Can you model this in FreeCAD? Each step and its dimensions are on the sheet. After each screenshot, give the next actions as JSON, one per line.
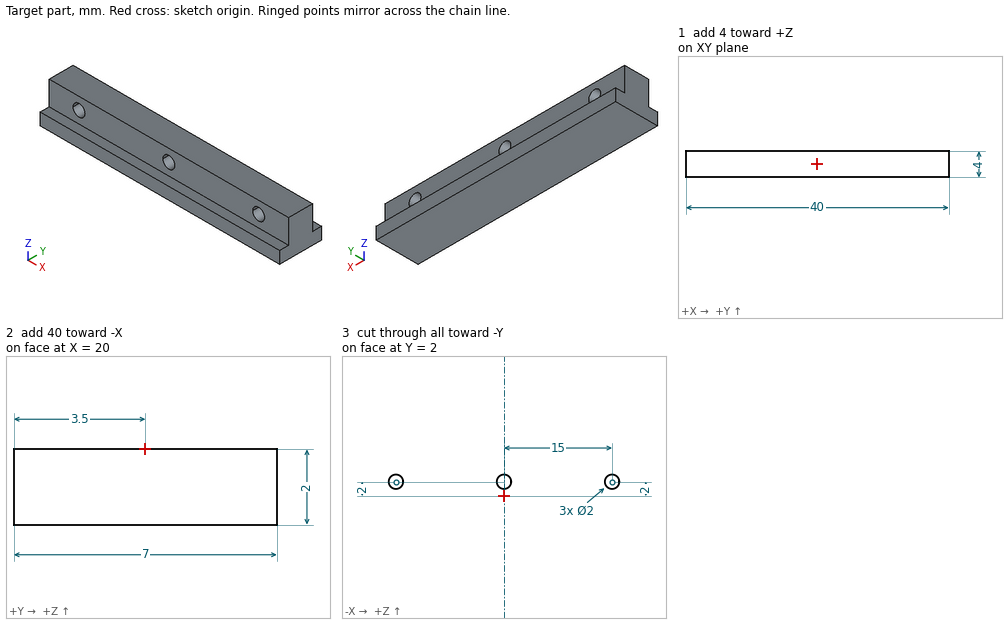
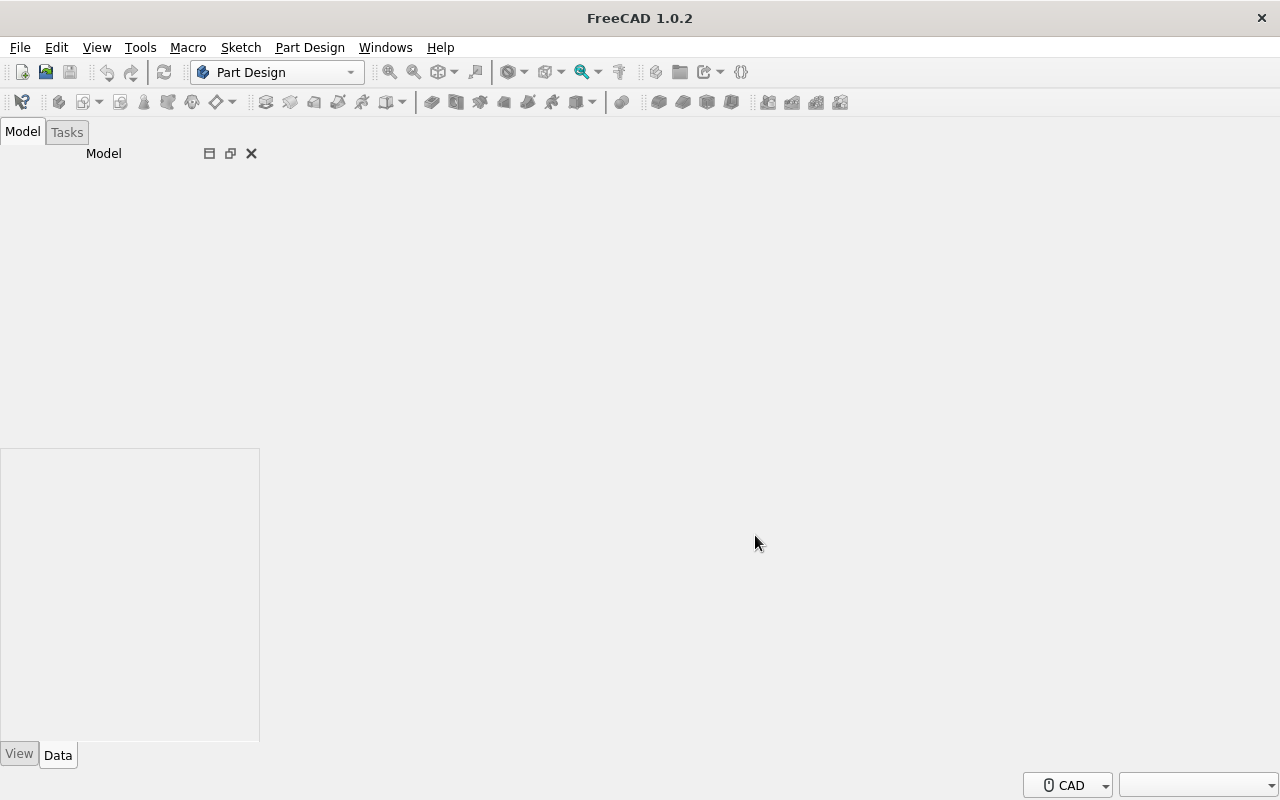
{"action": "key", "text": "ctrl+n"}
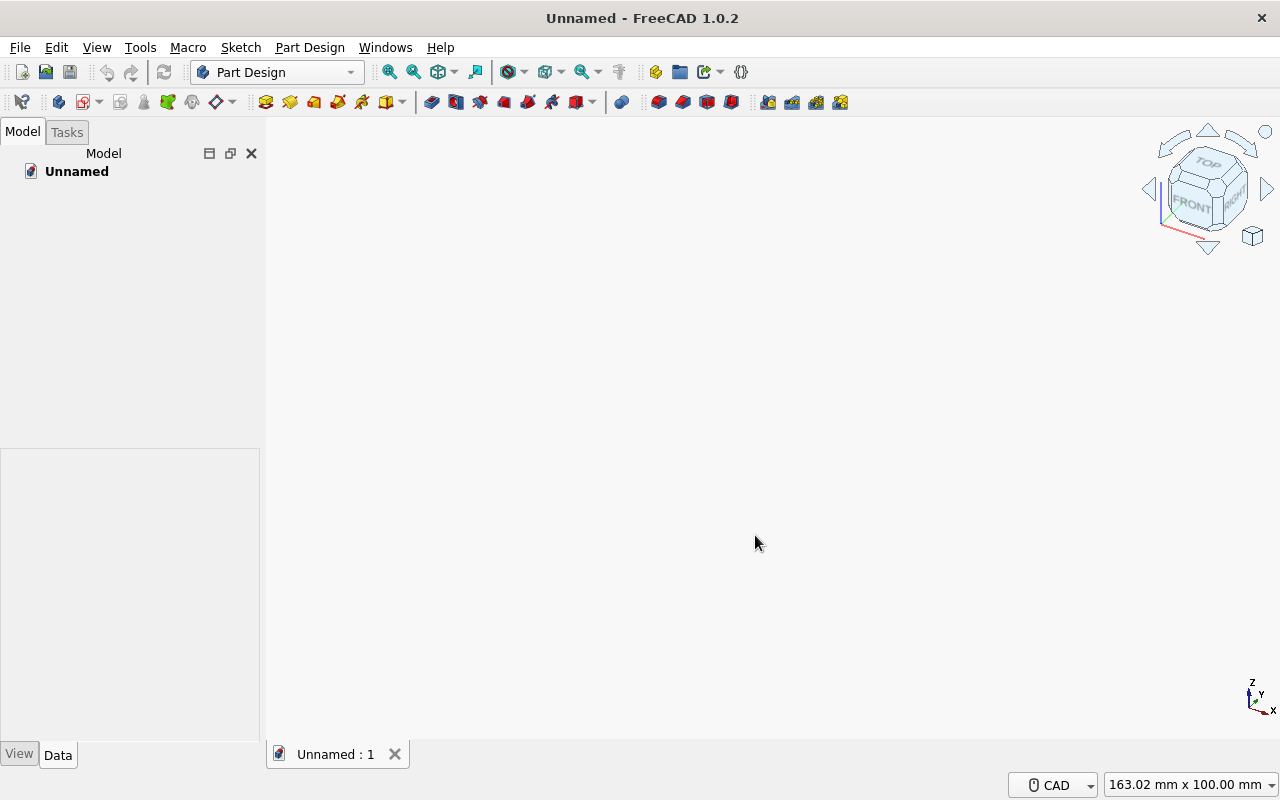
{"action": "left_click", "coordinate": [84, 102]}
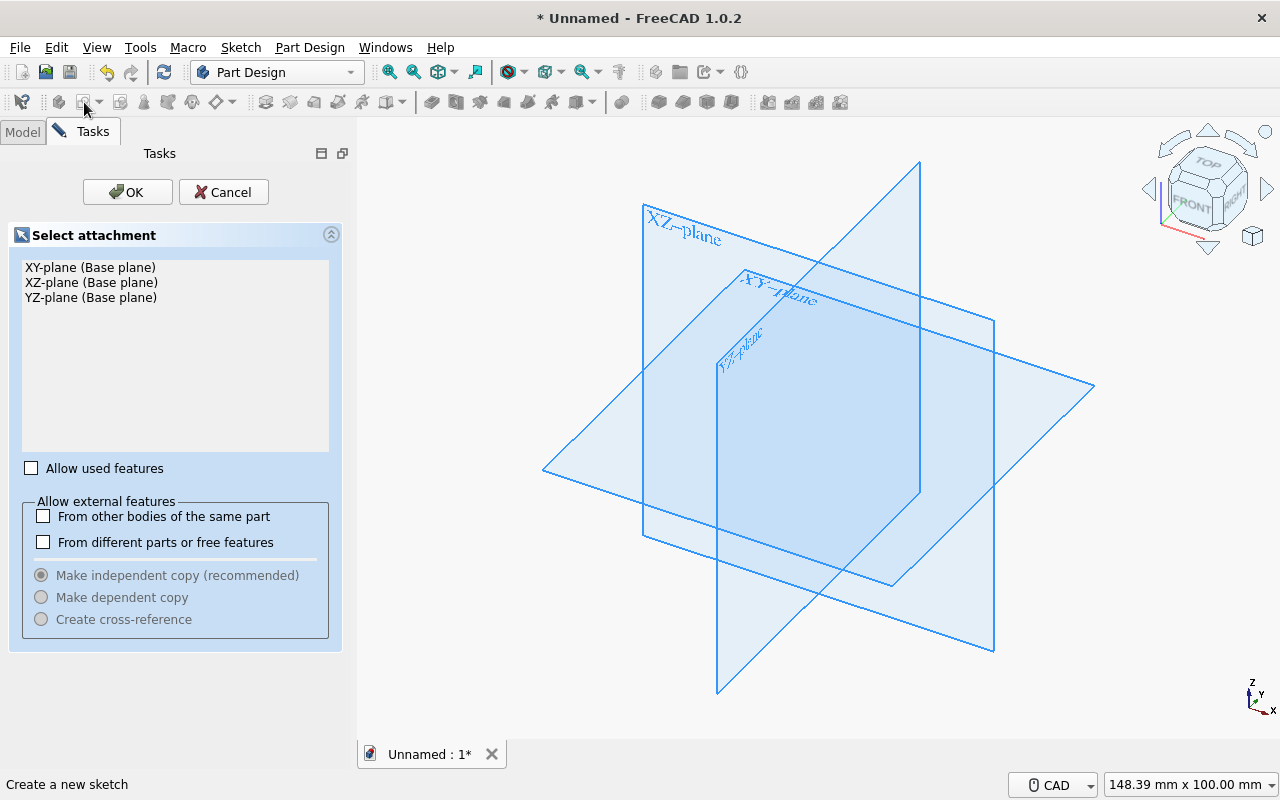
{"action": "left_click", "coordinate": [82, 268]}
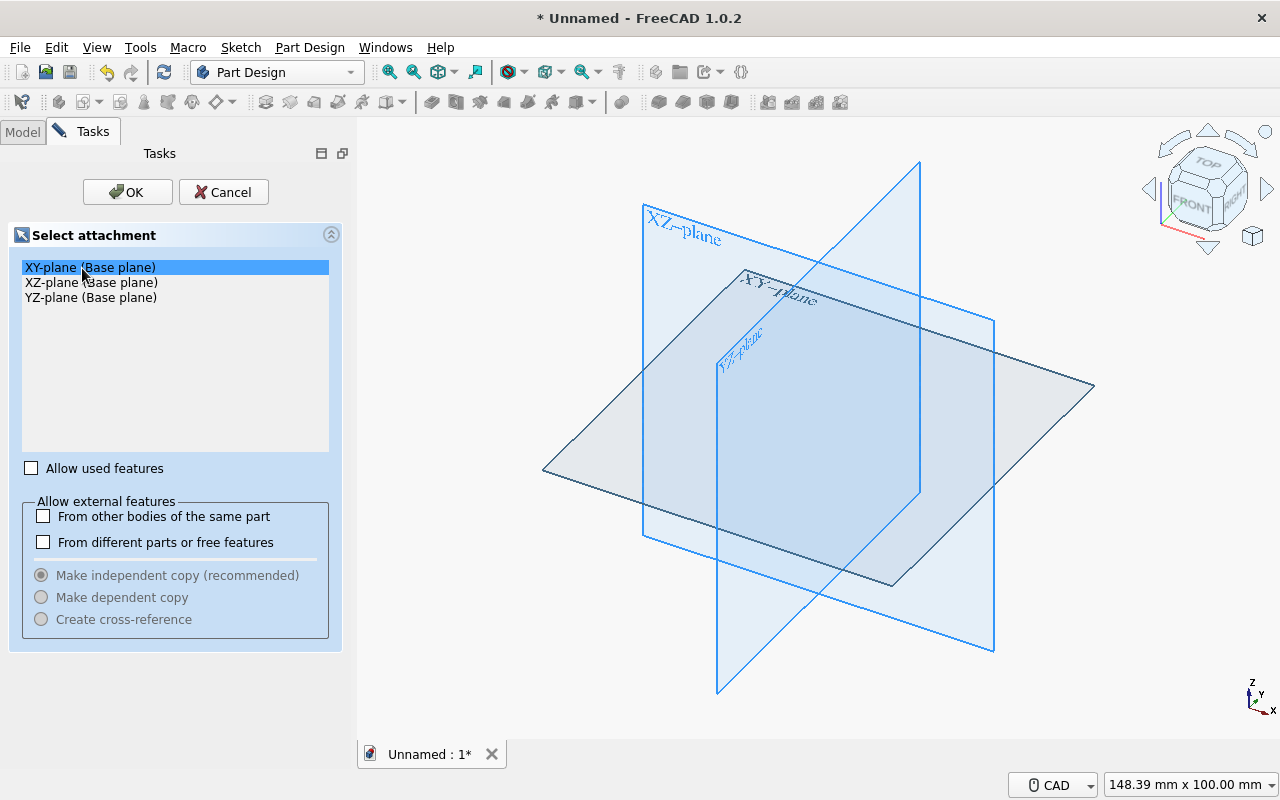
{"action": "left_click", "coordinate": [128, 192]}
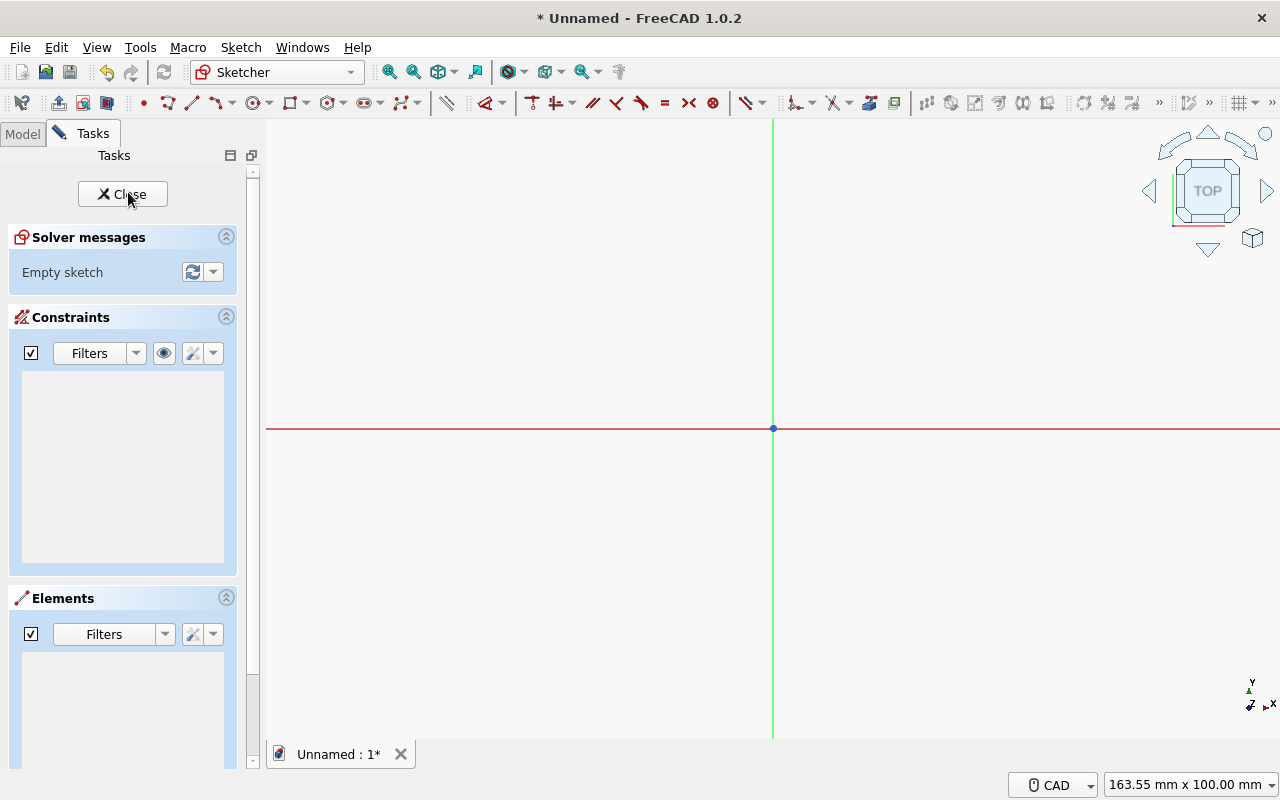
{"action": "scroll", "coordinate": [829, 429], "scroll_direction": "up", "scroll_amount": 4}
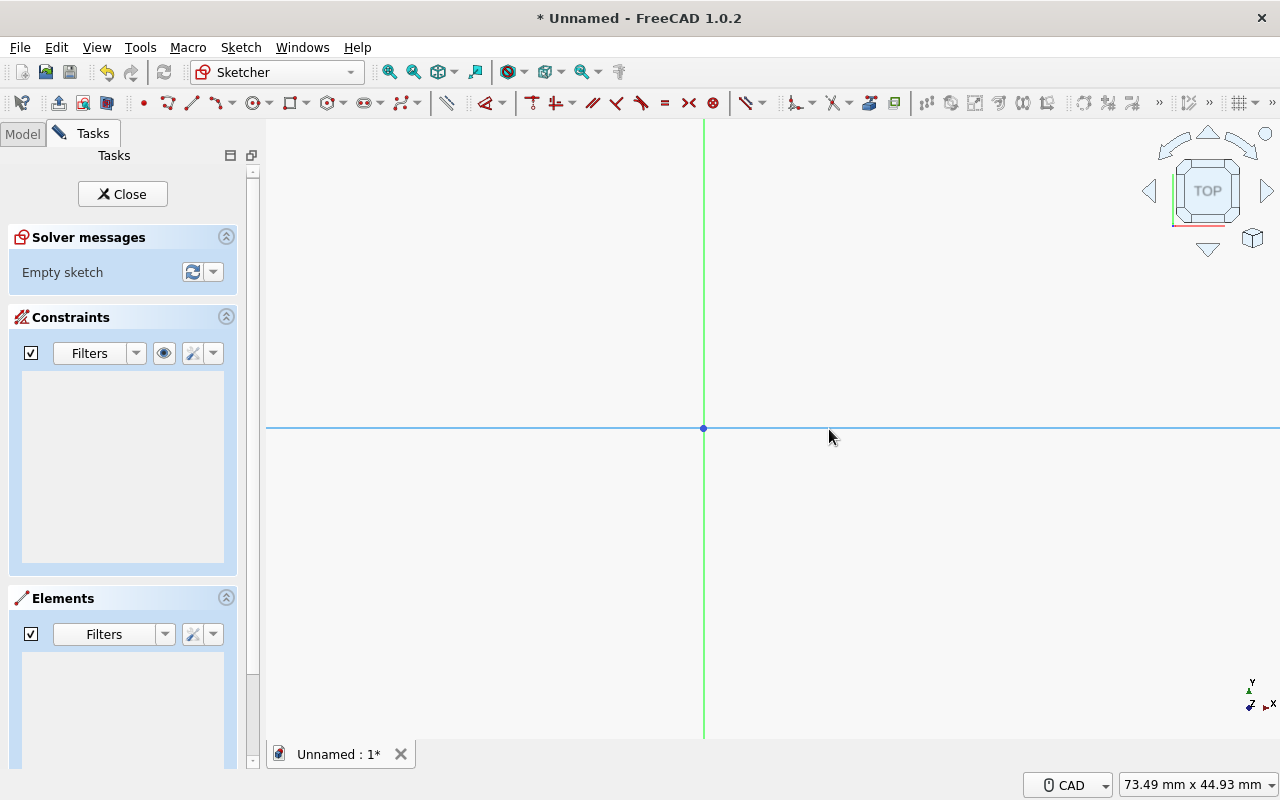
{"action": "left_click", "coordinate": [308, 104]}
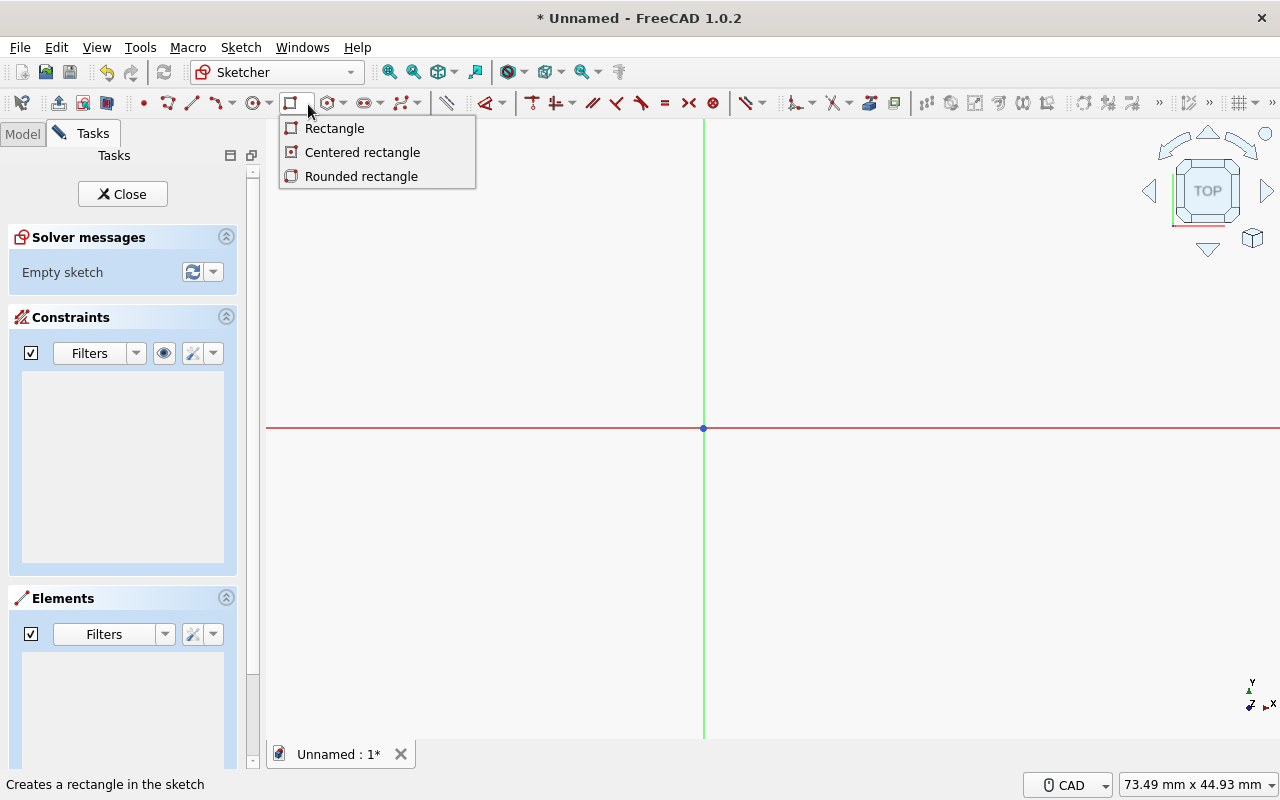
{"action": "left_click", "coordinate": [378, 152]}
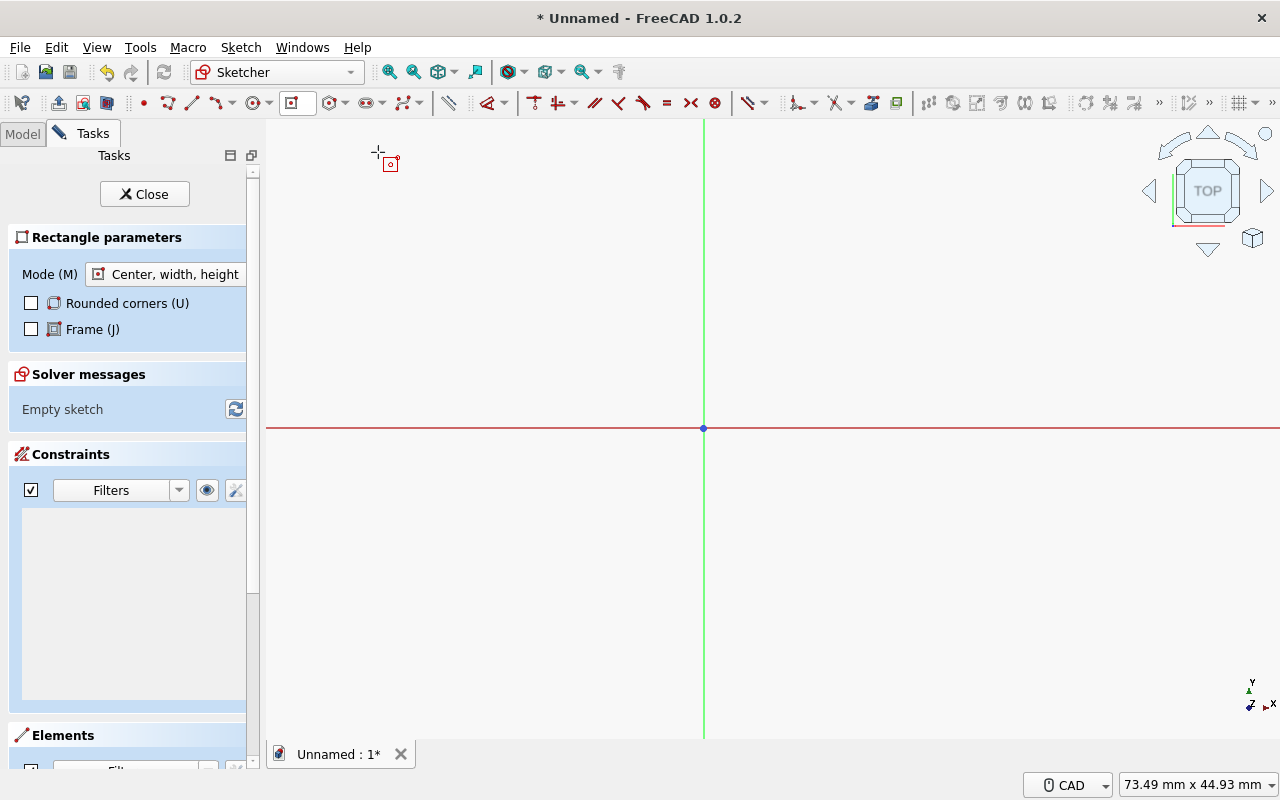
{"action": "left_click", "coordinate": [704, 428]}
{"action": "mouse_move", "coordinate": [980, 401]}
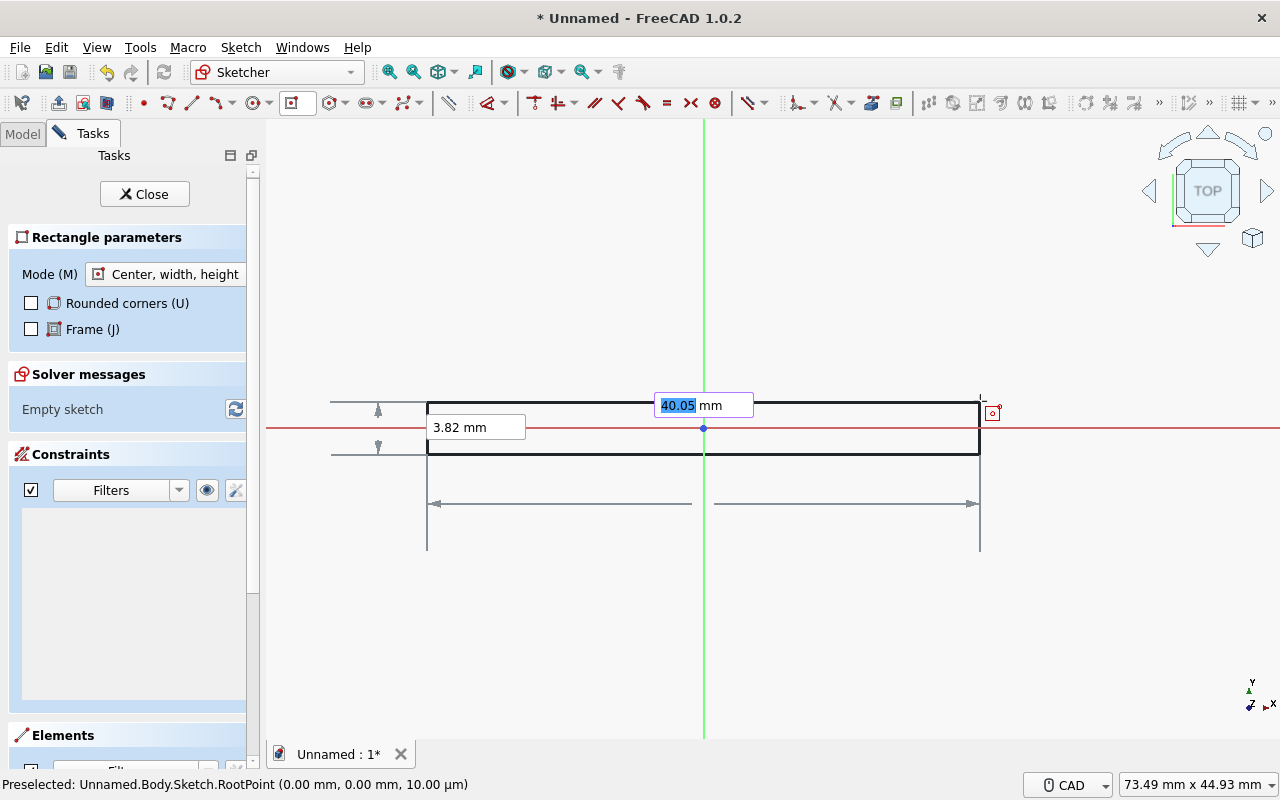
{"action": "type", "text": "40"}
{"action": "key", "text": "Tab"}
{"action": "type", "text": "4"}
{"action": "key", "text": "Return"}
{"action": "key", "text": "Escape"}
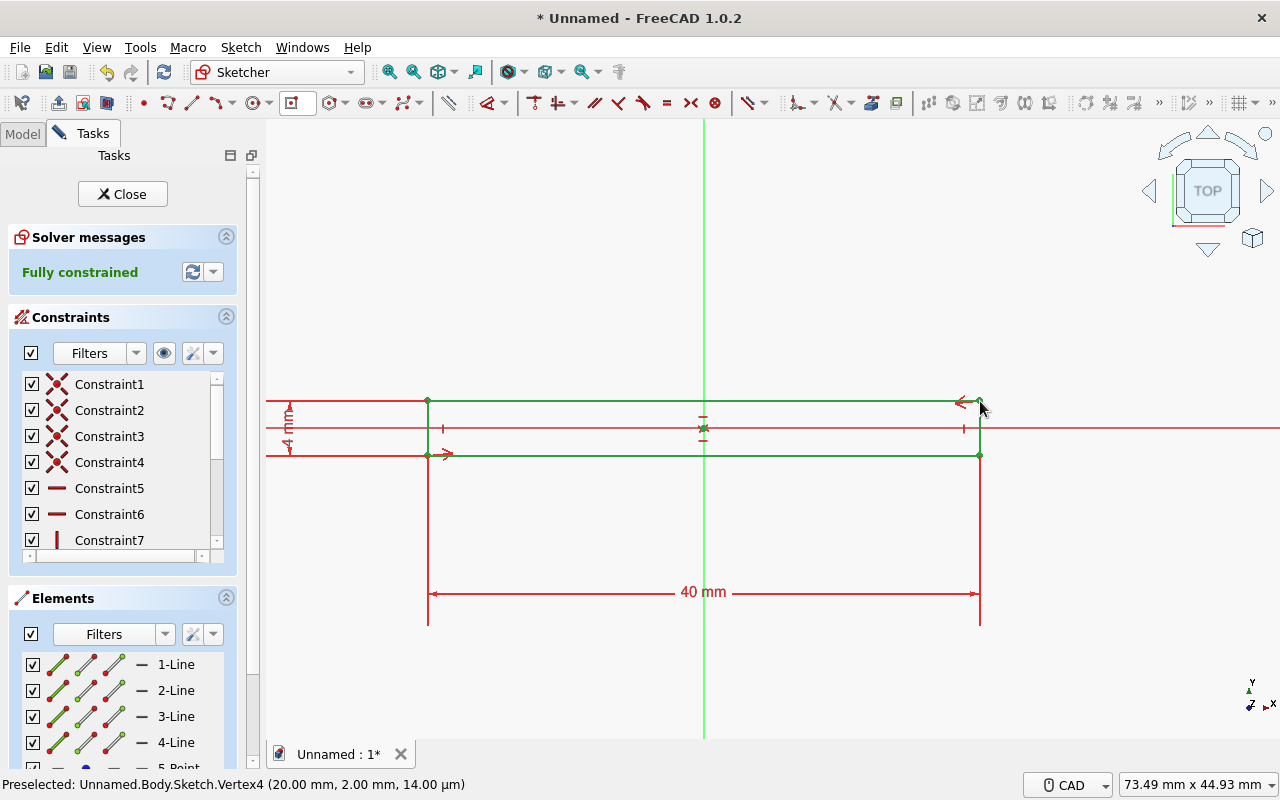
{"action": "left_click", "coordinate": [123, 194]}